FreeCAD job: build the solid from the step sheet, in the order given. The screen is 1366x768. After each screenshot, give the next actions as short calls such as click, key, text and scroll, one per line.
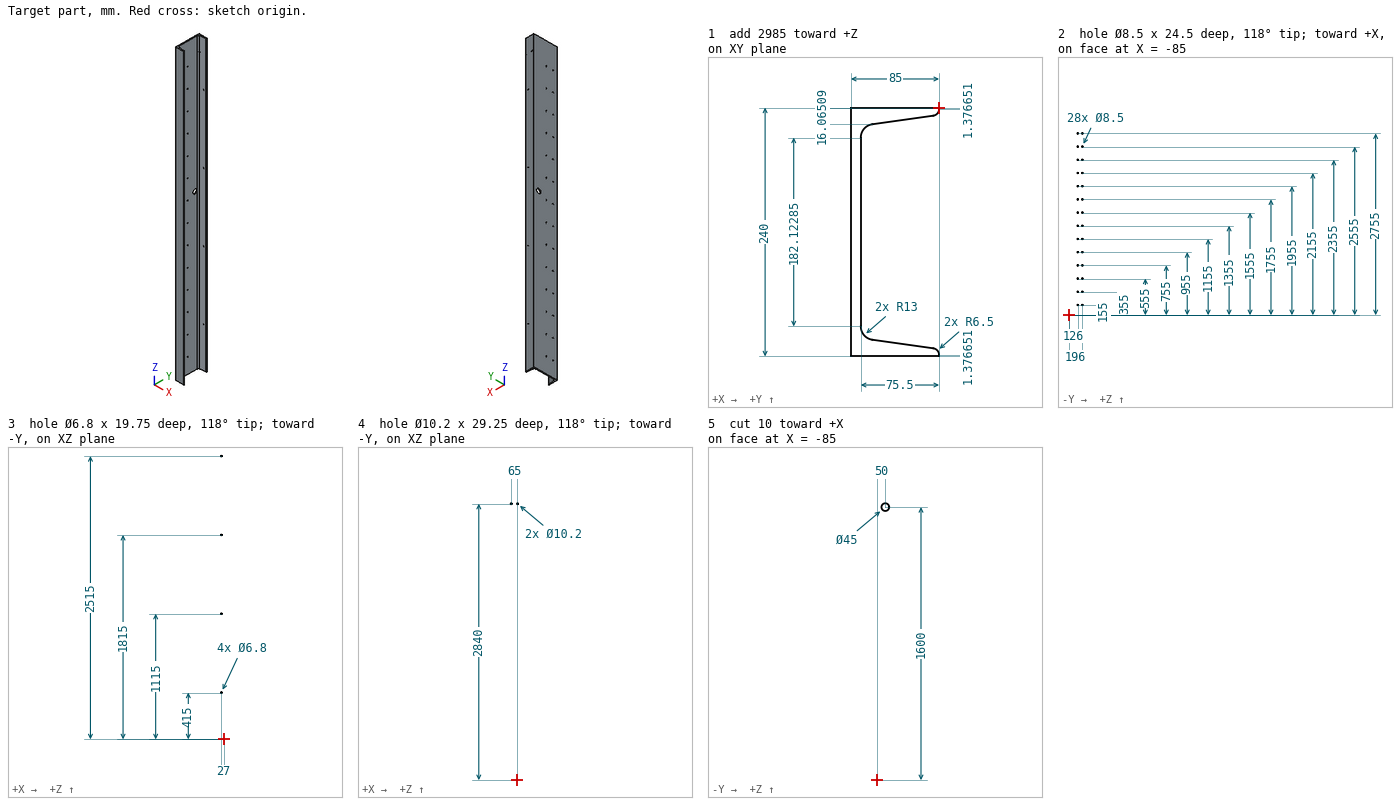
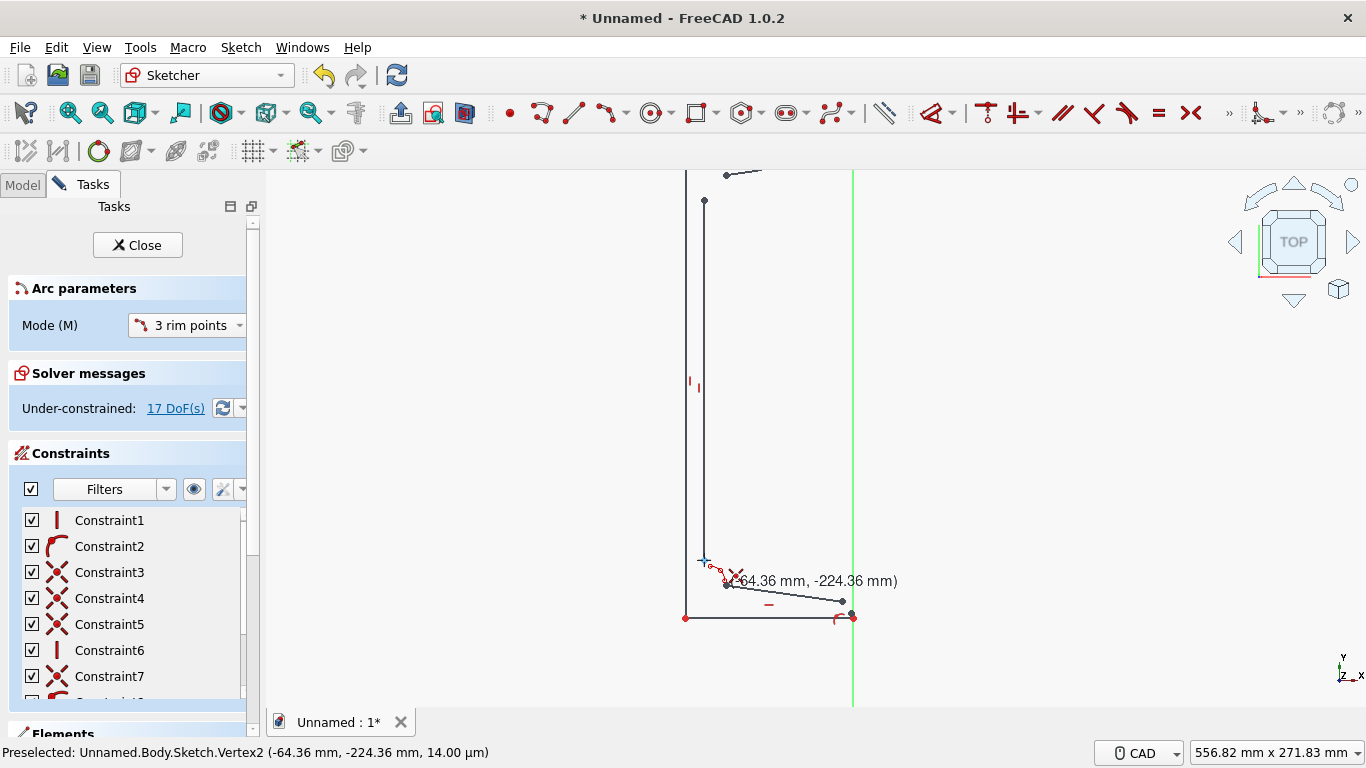
click(704, 560)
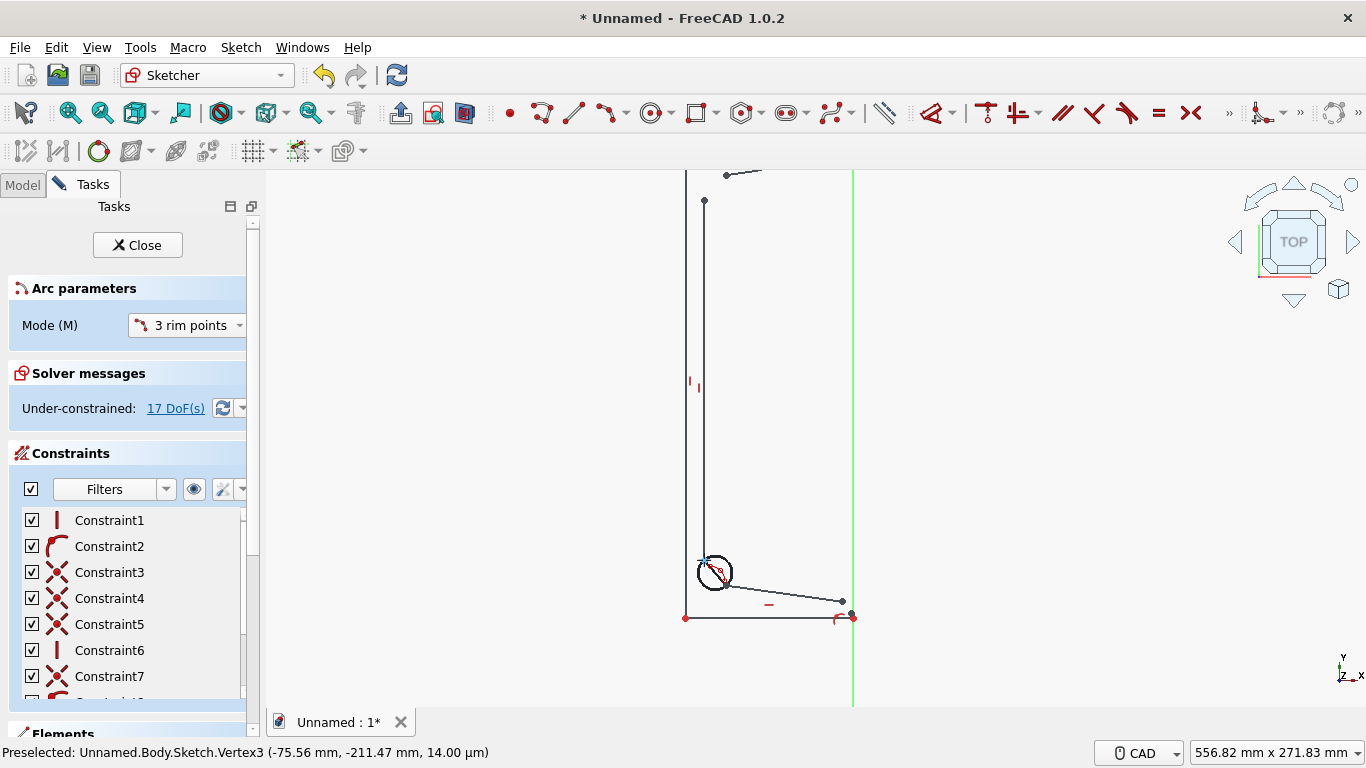
scroll(710, 576, up, 5)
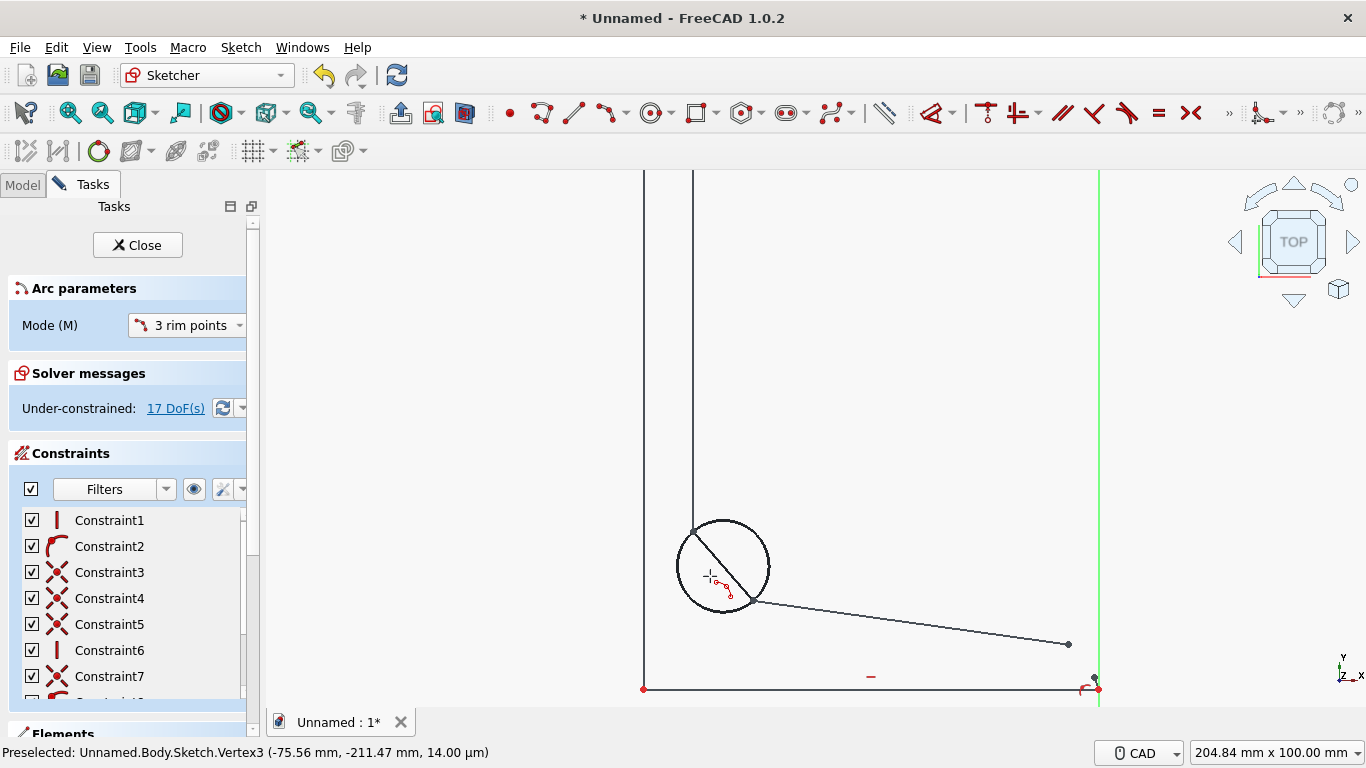
click(711, 575)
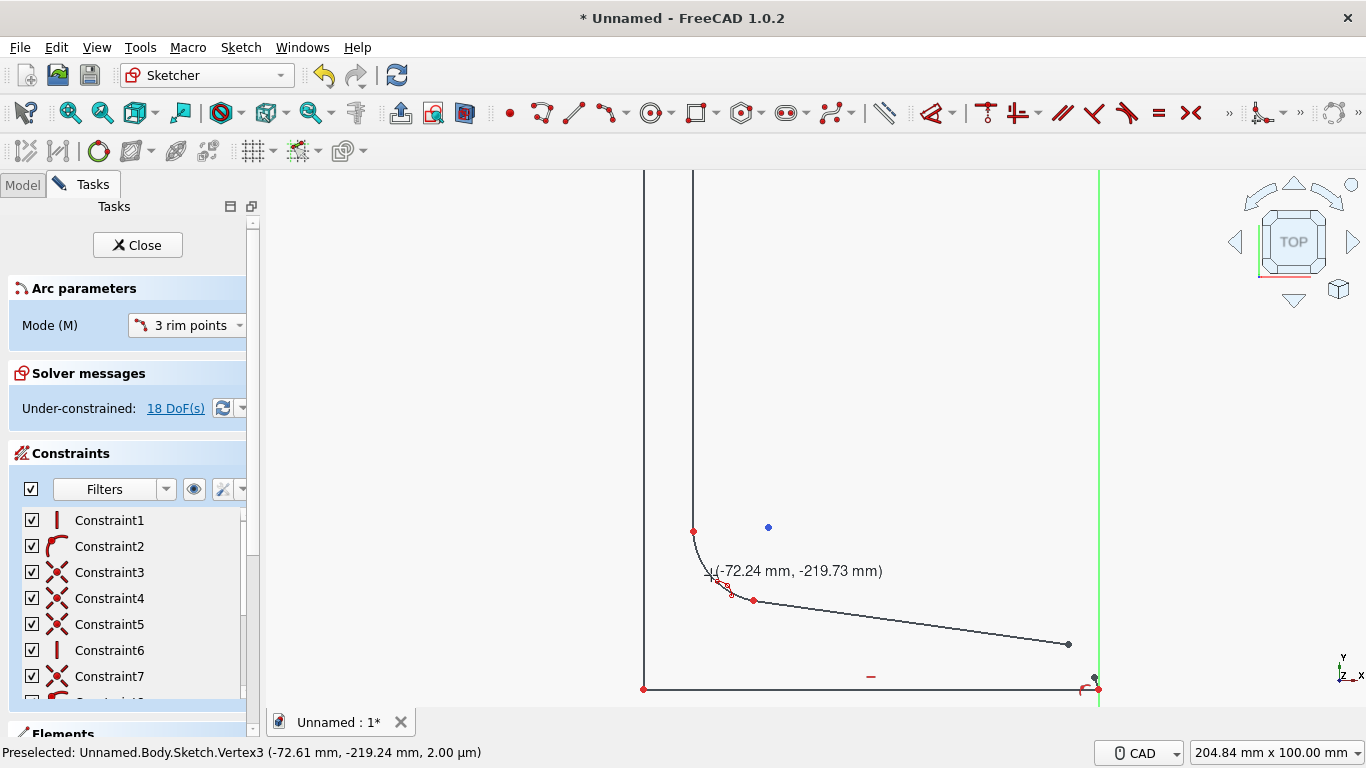
scroll(707, 569, down, 7)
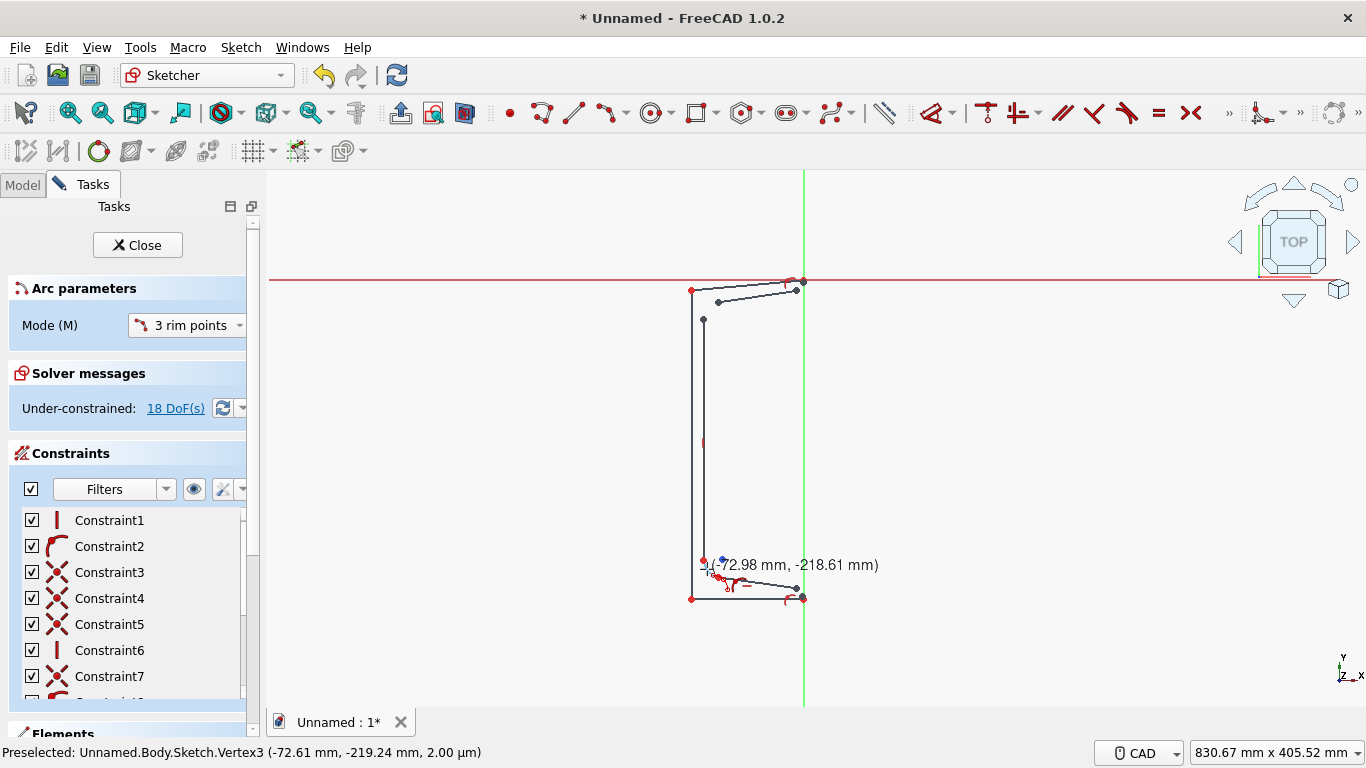
scroll(704, 319, up, 2)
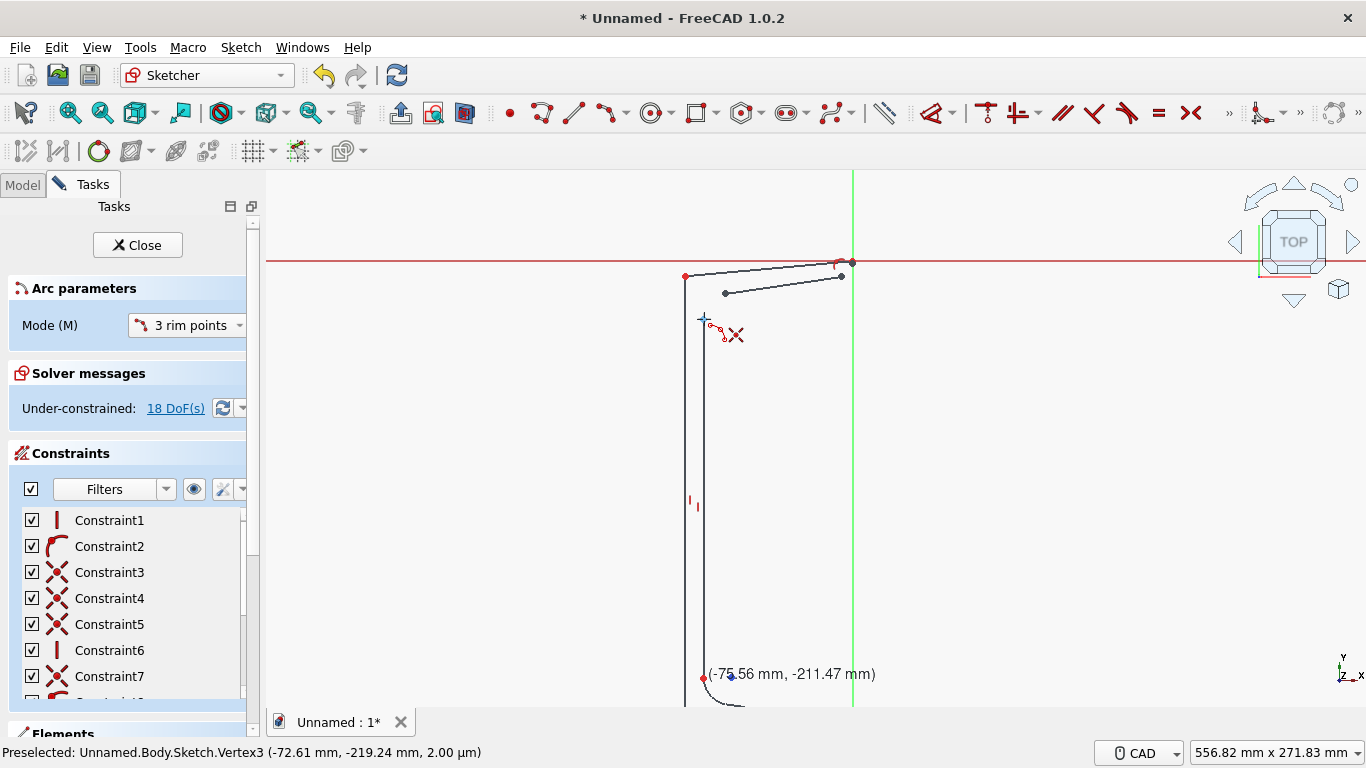
click(704, 319)
click(726, 294)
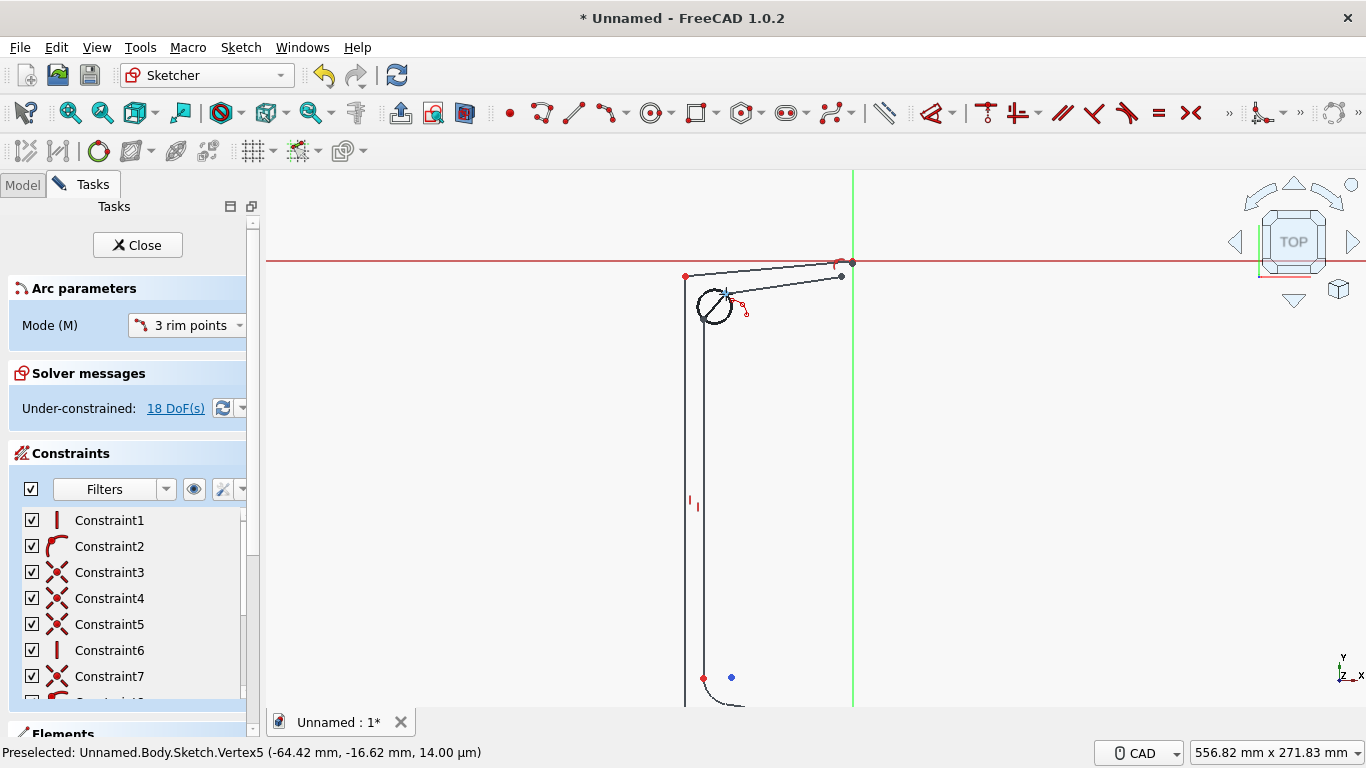
scroll(710, 301, up, 5)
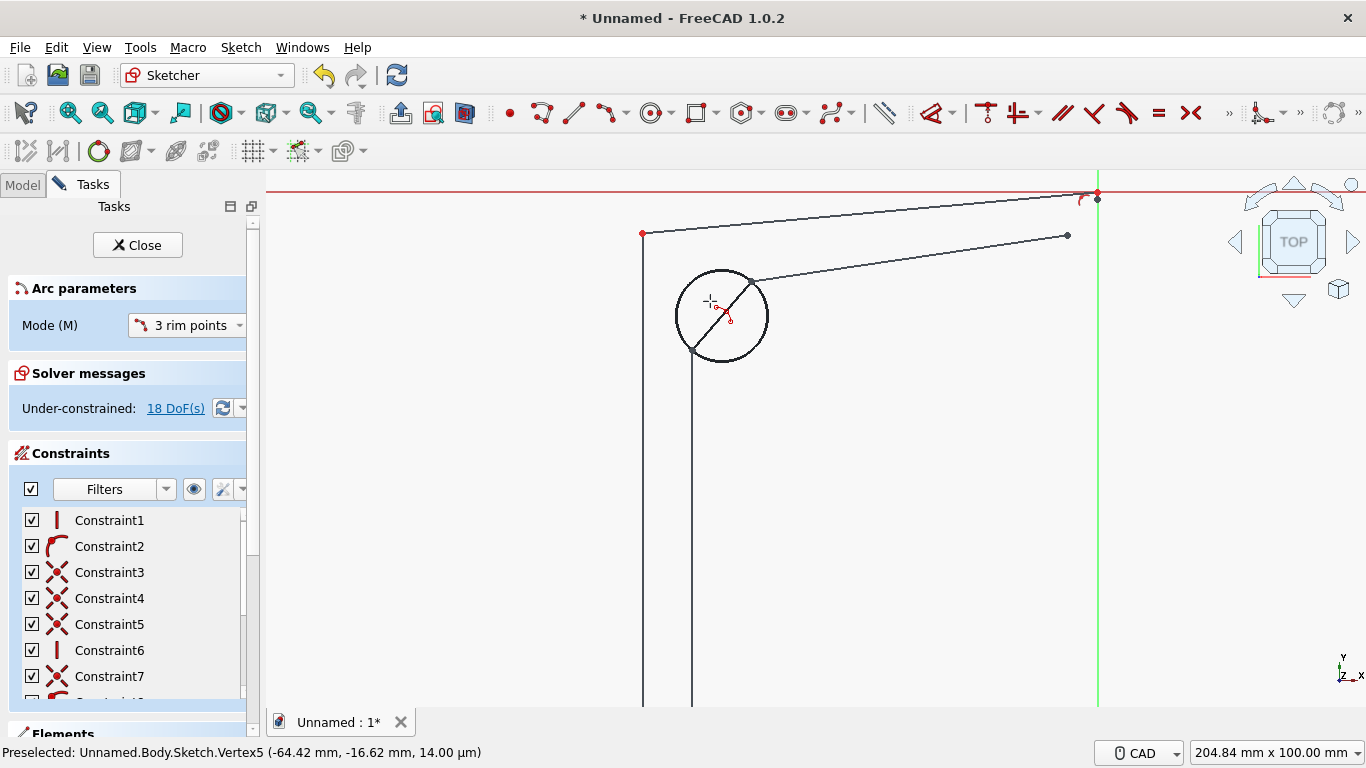
click(709, 302)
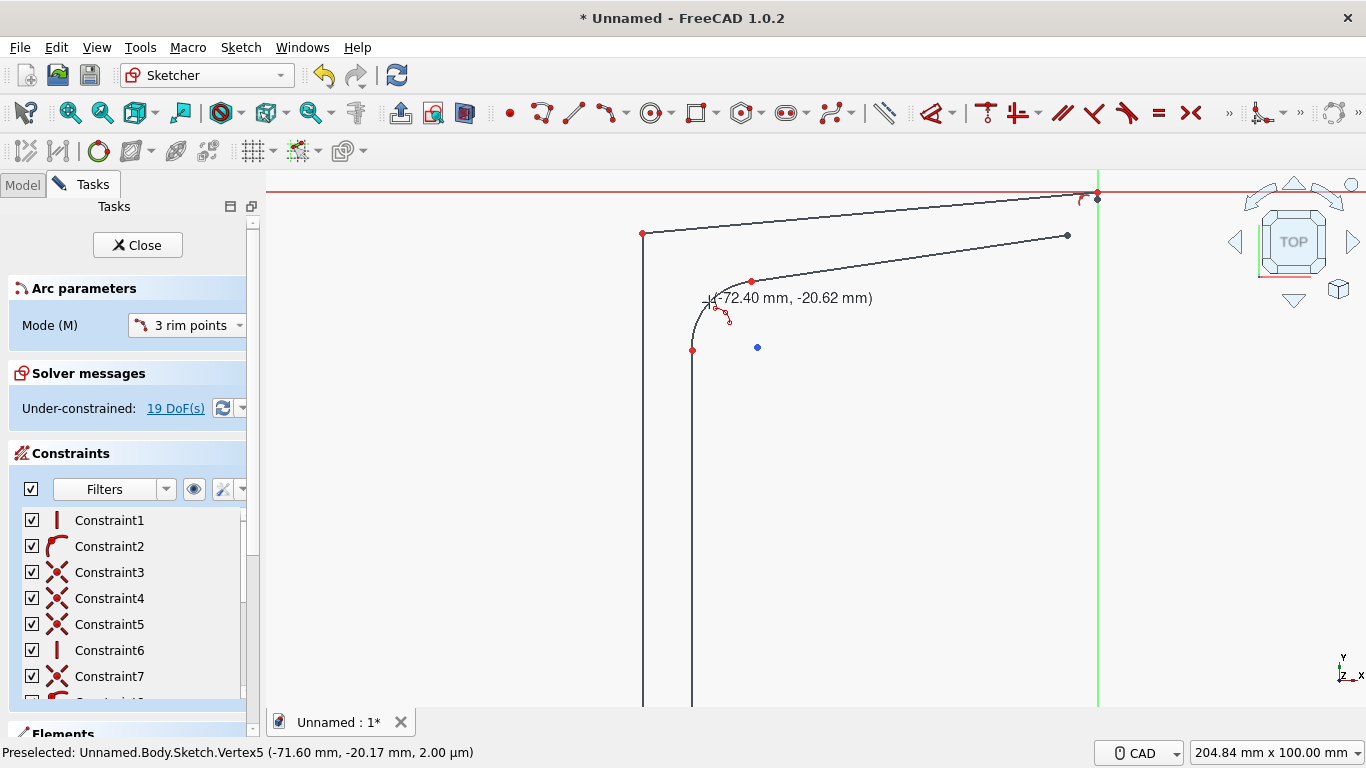
click(1067, 235)